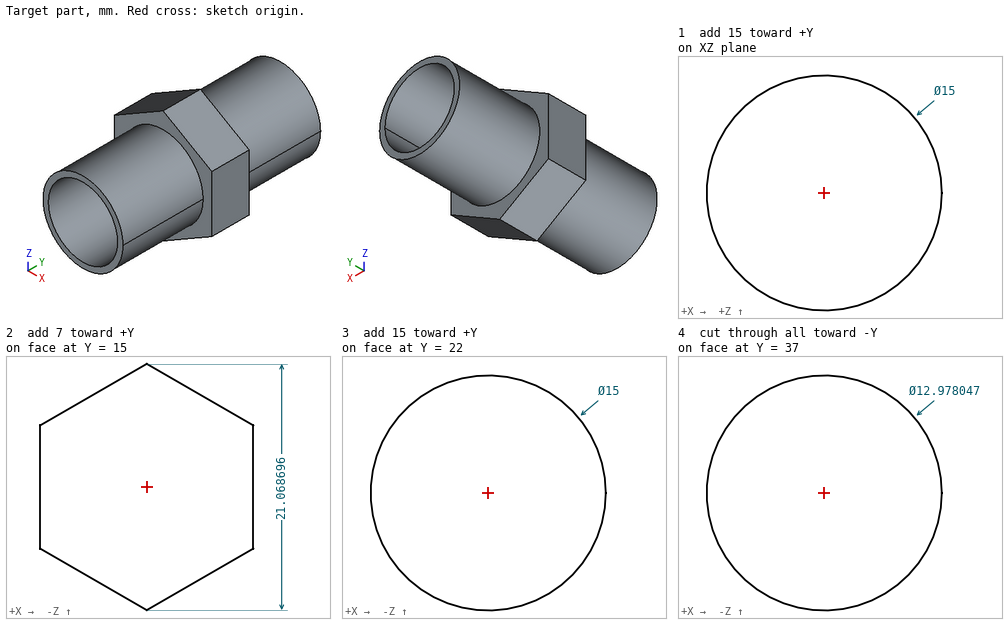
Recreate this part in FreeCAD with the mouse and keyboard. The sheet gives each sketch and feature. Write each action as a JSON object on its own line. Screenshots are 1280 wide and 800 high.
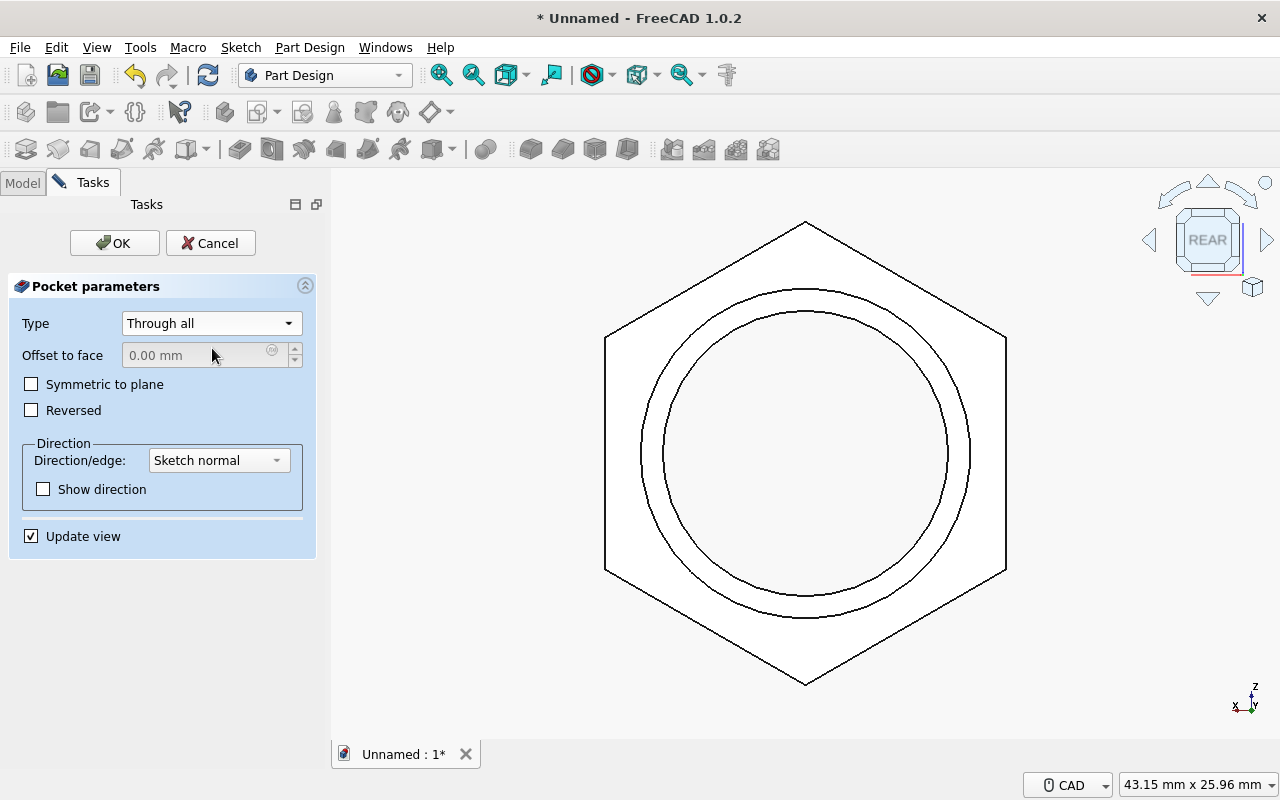
{"action": "left_click", "coordinate": [115, 243]}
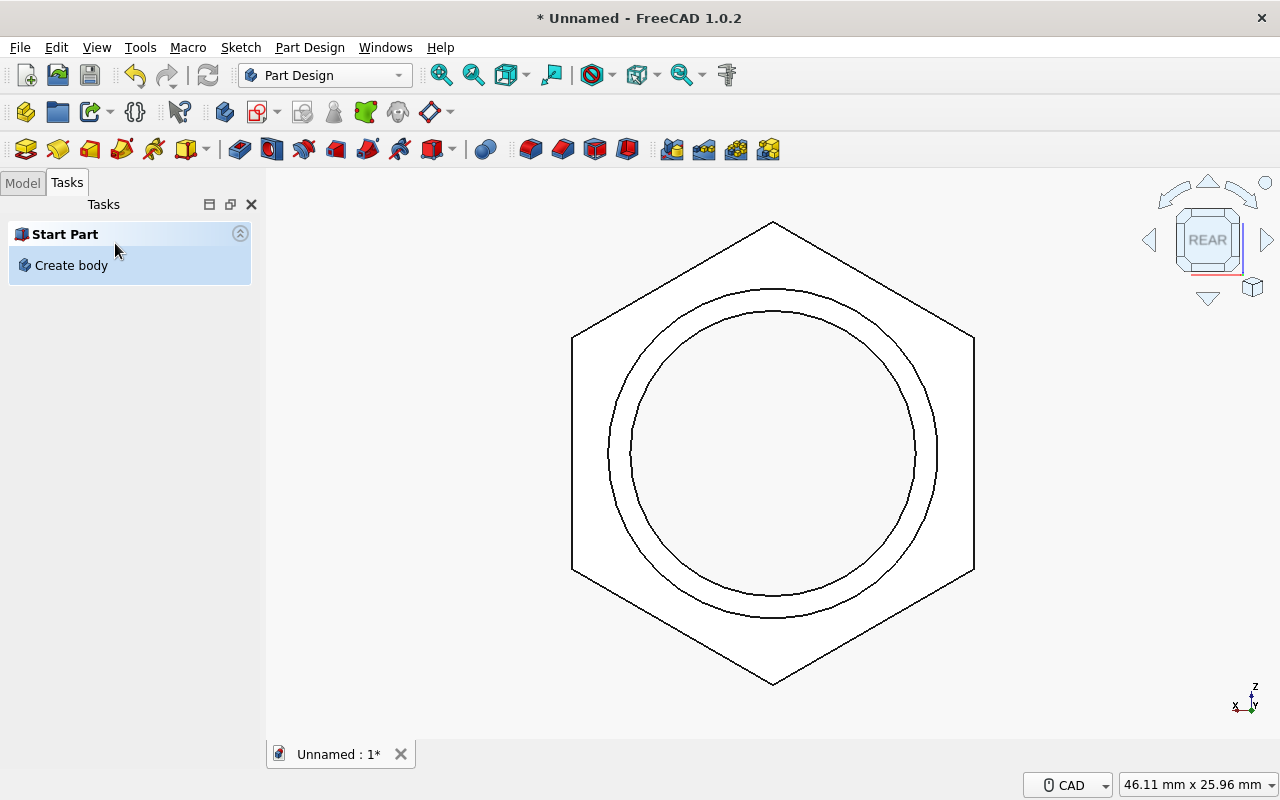
{"action": "key", "text": "0"}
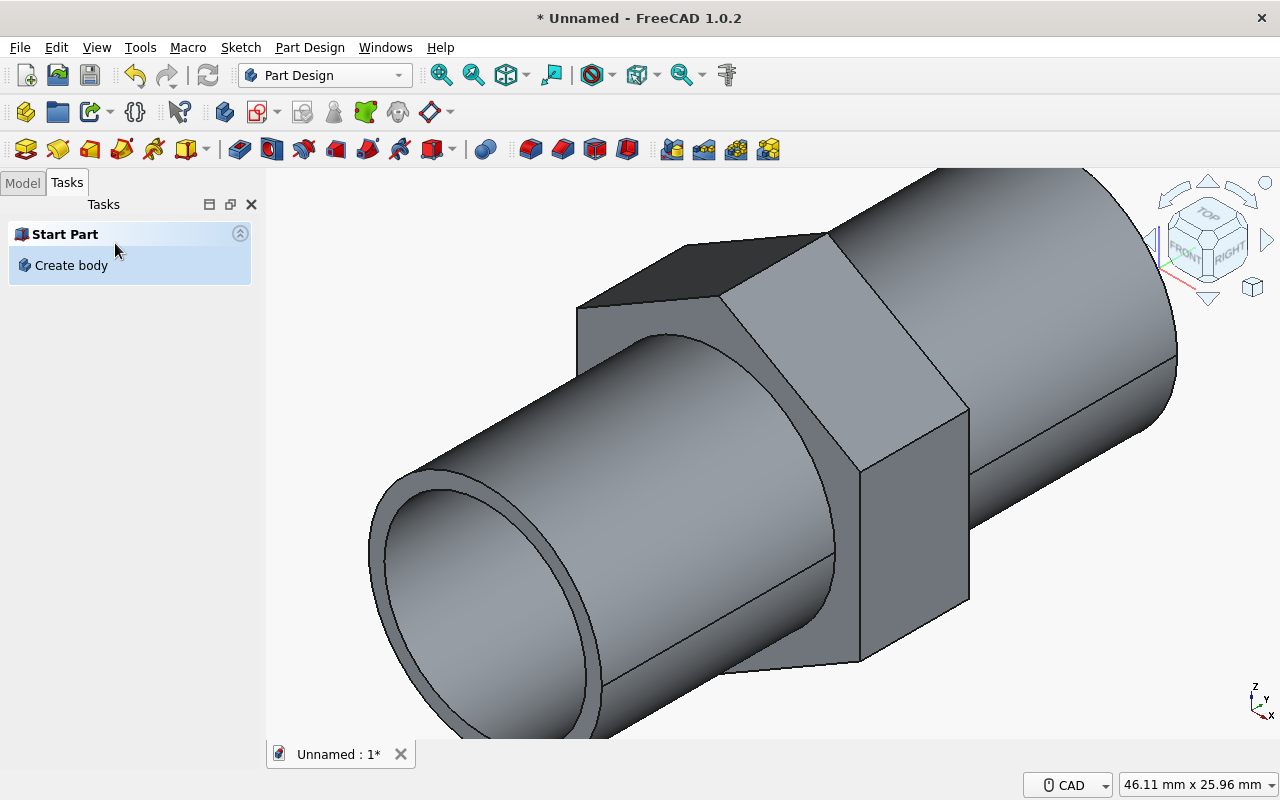
{"action": "left_click", "coordinate": [442, 76]}